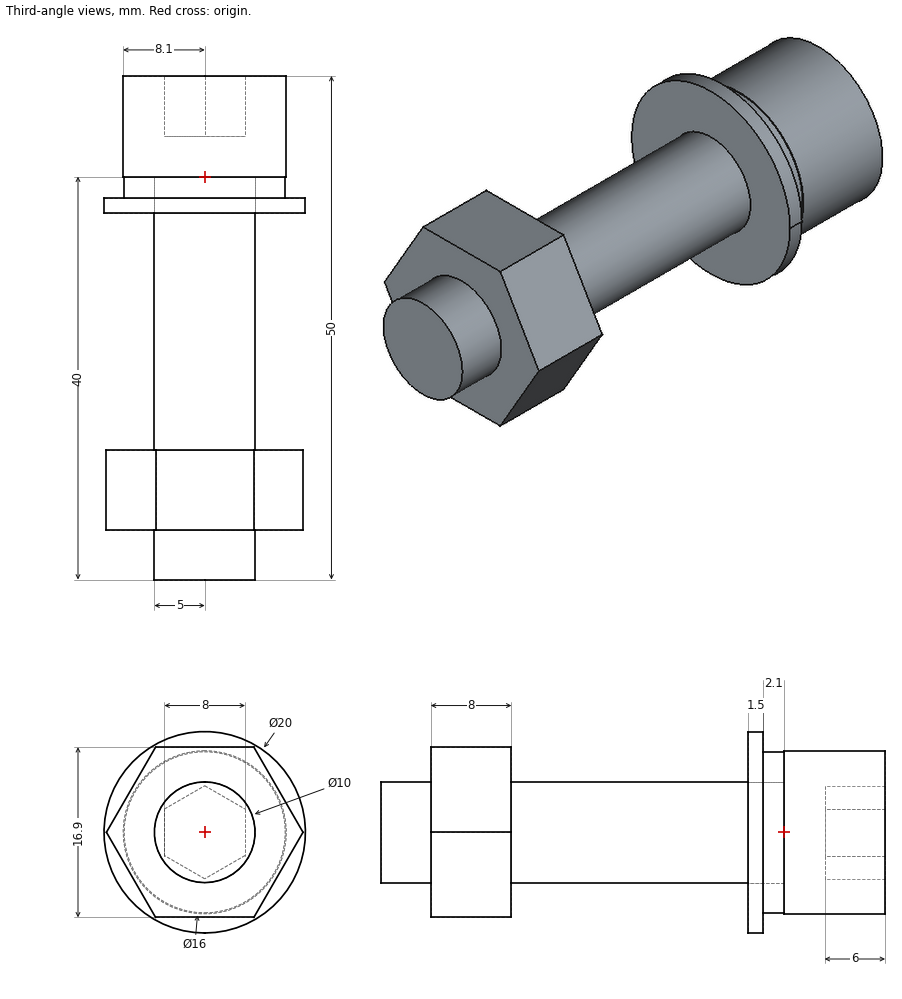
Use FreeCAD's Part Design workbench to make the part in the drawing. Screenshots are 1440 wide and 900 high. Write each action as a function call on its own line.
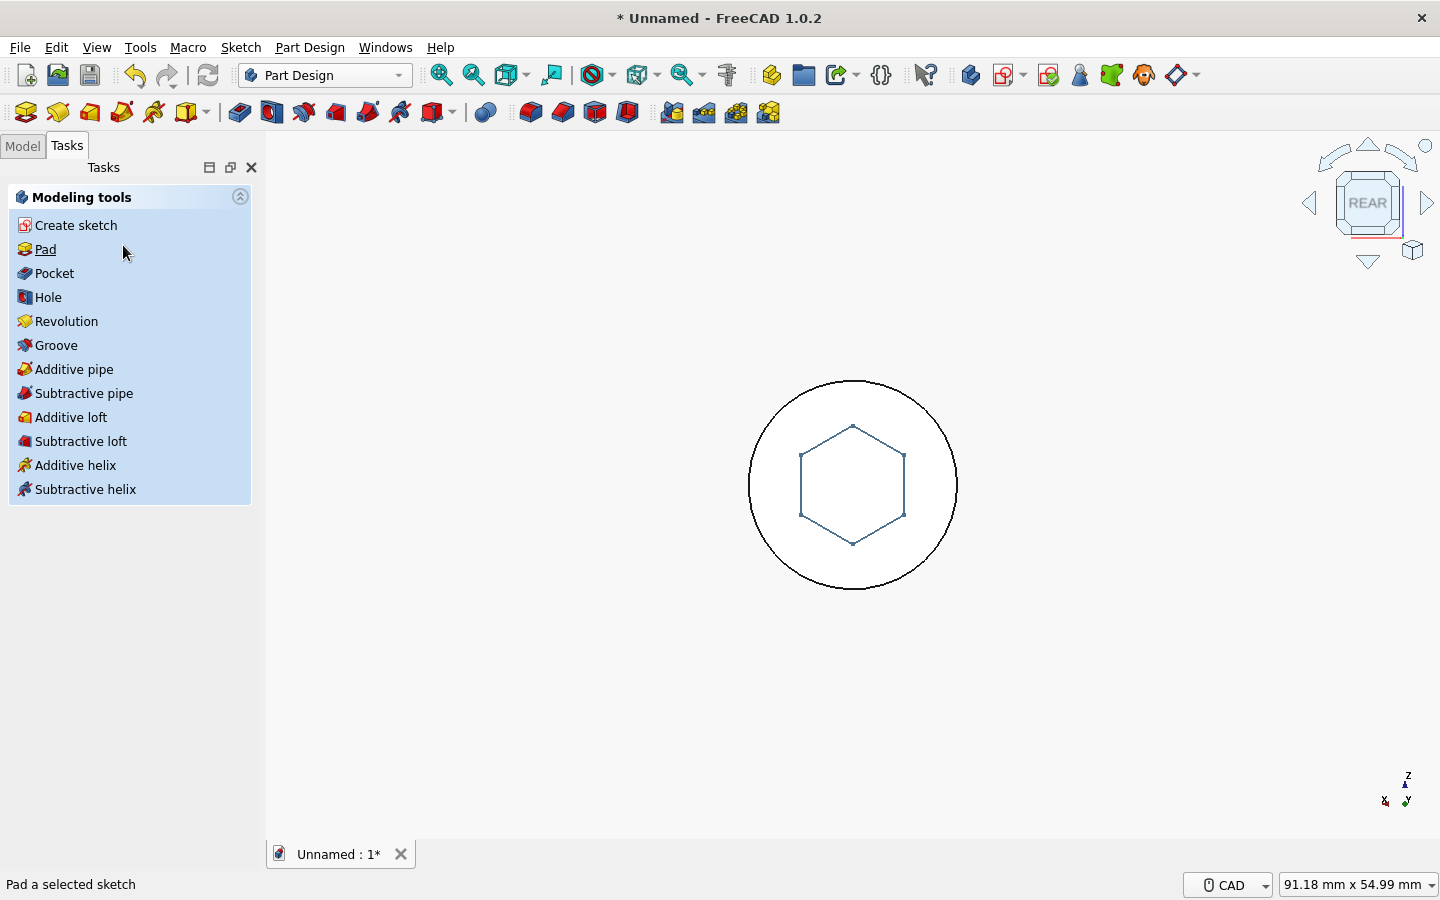
click(240, 112)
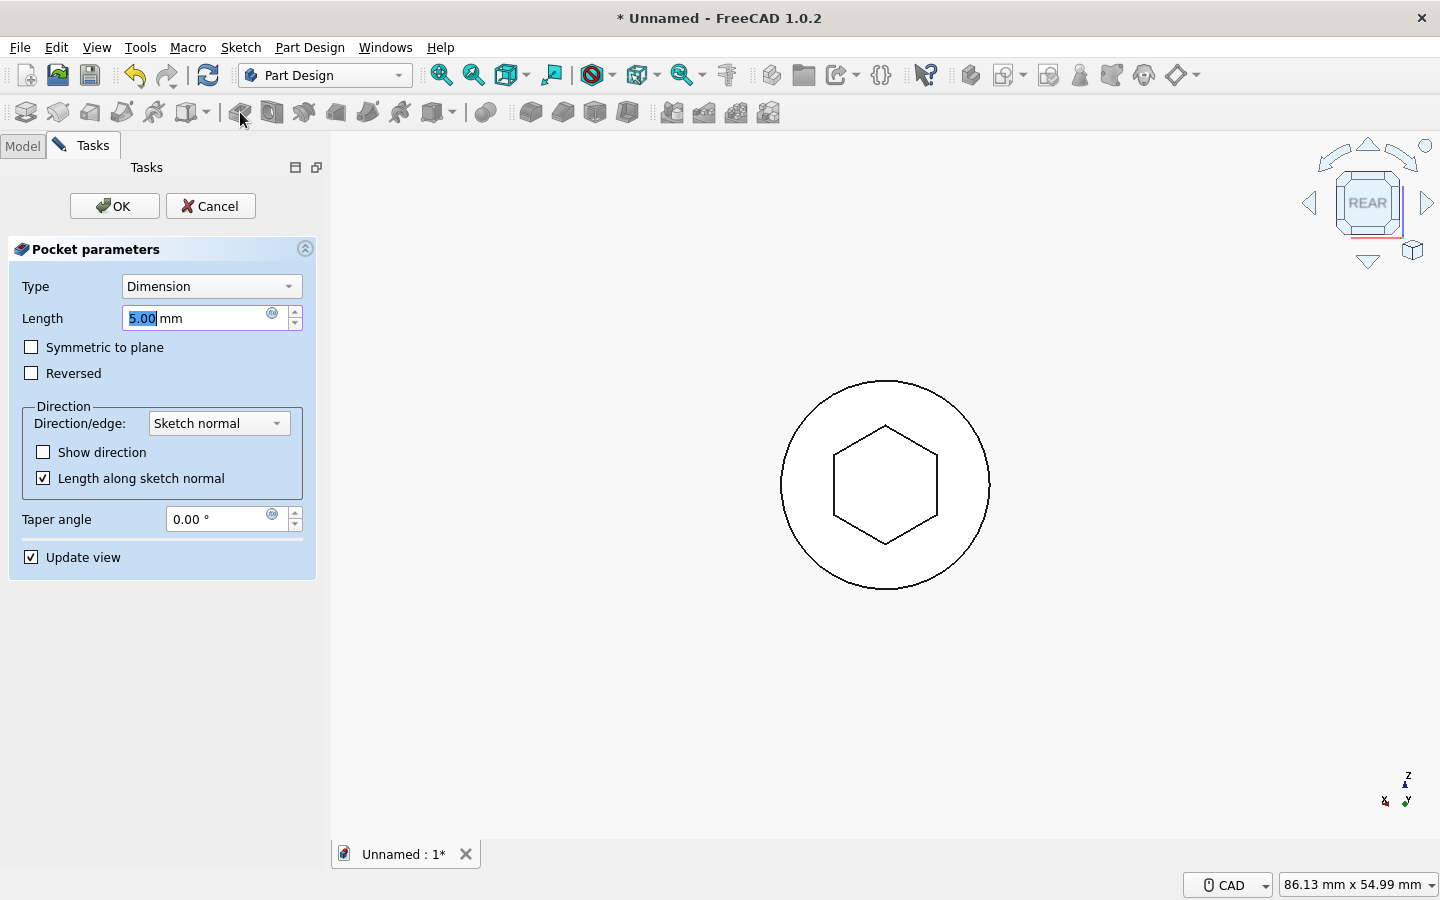
text(6)
key(Tab)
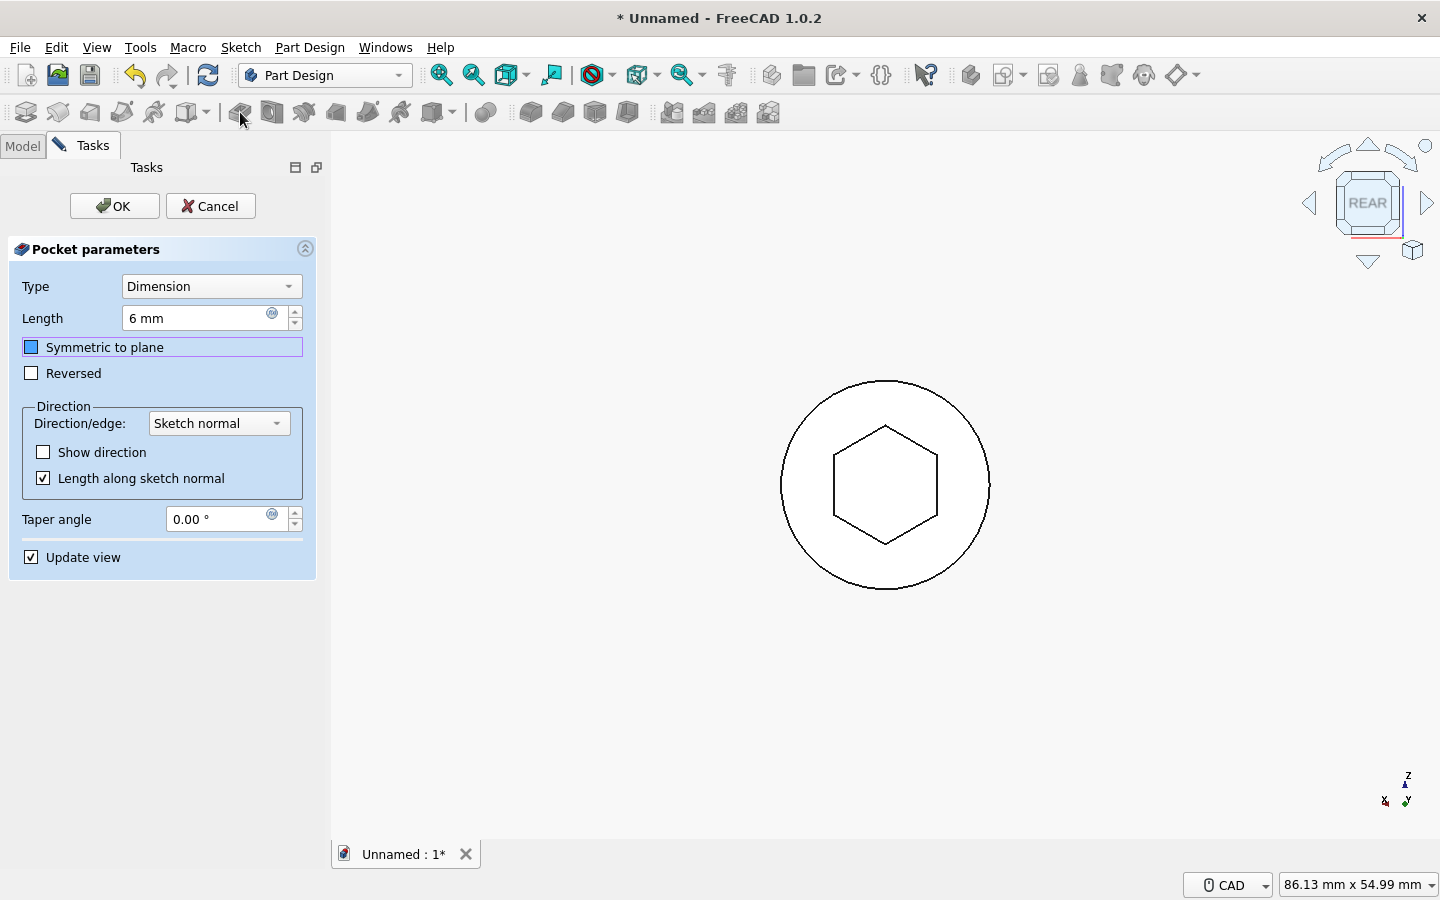
click(115, 206)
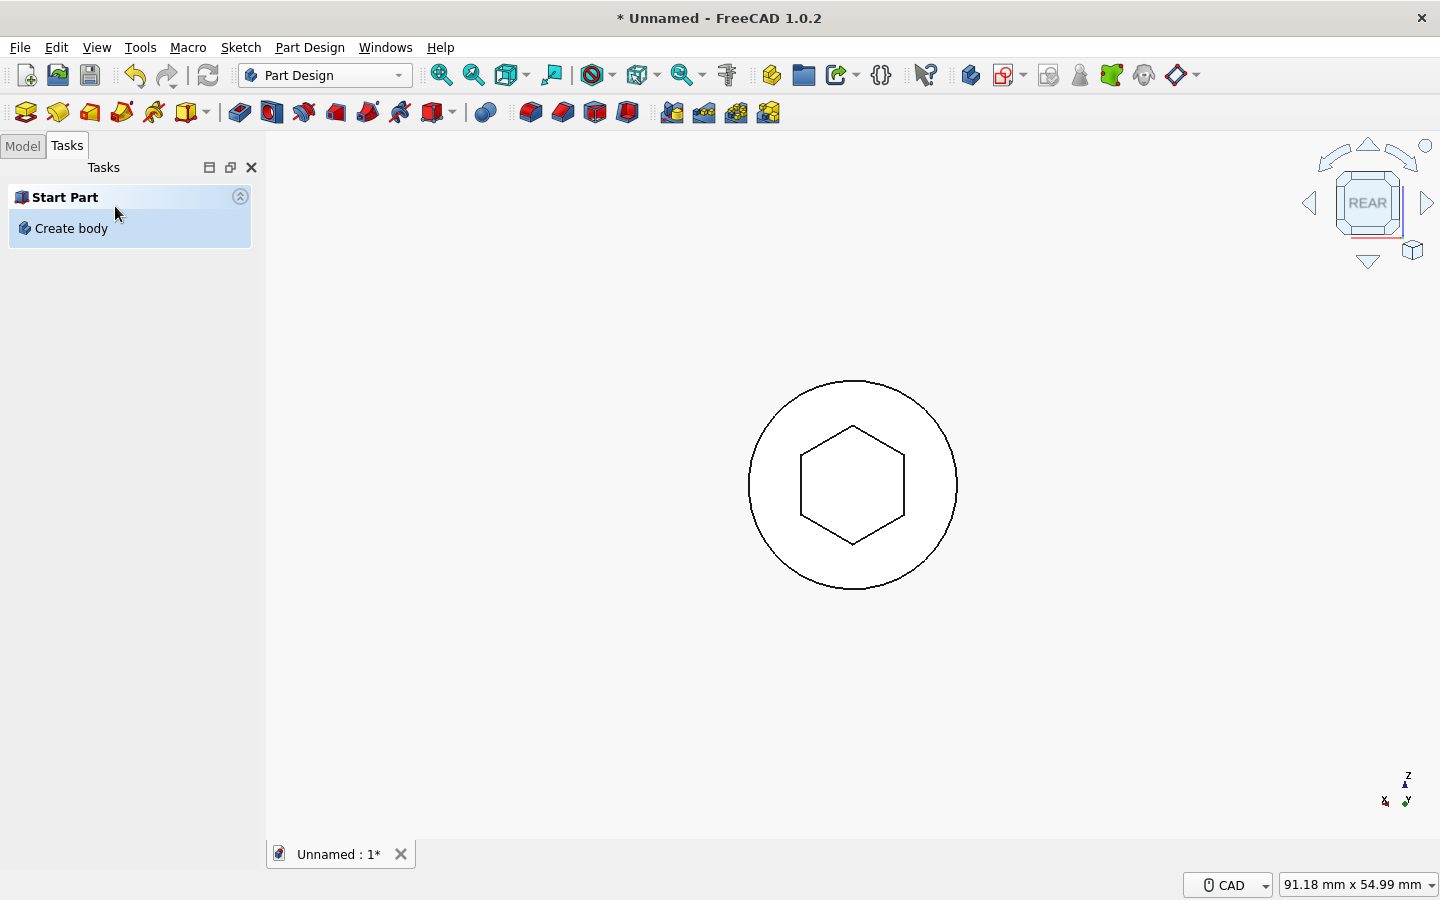
click(442, 76)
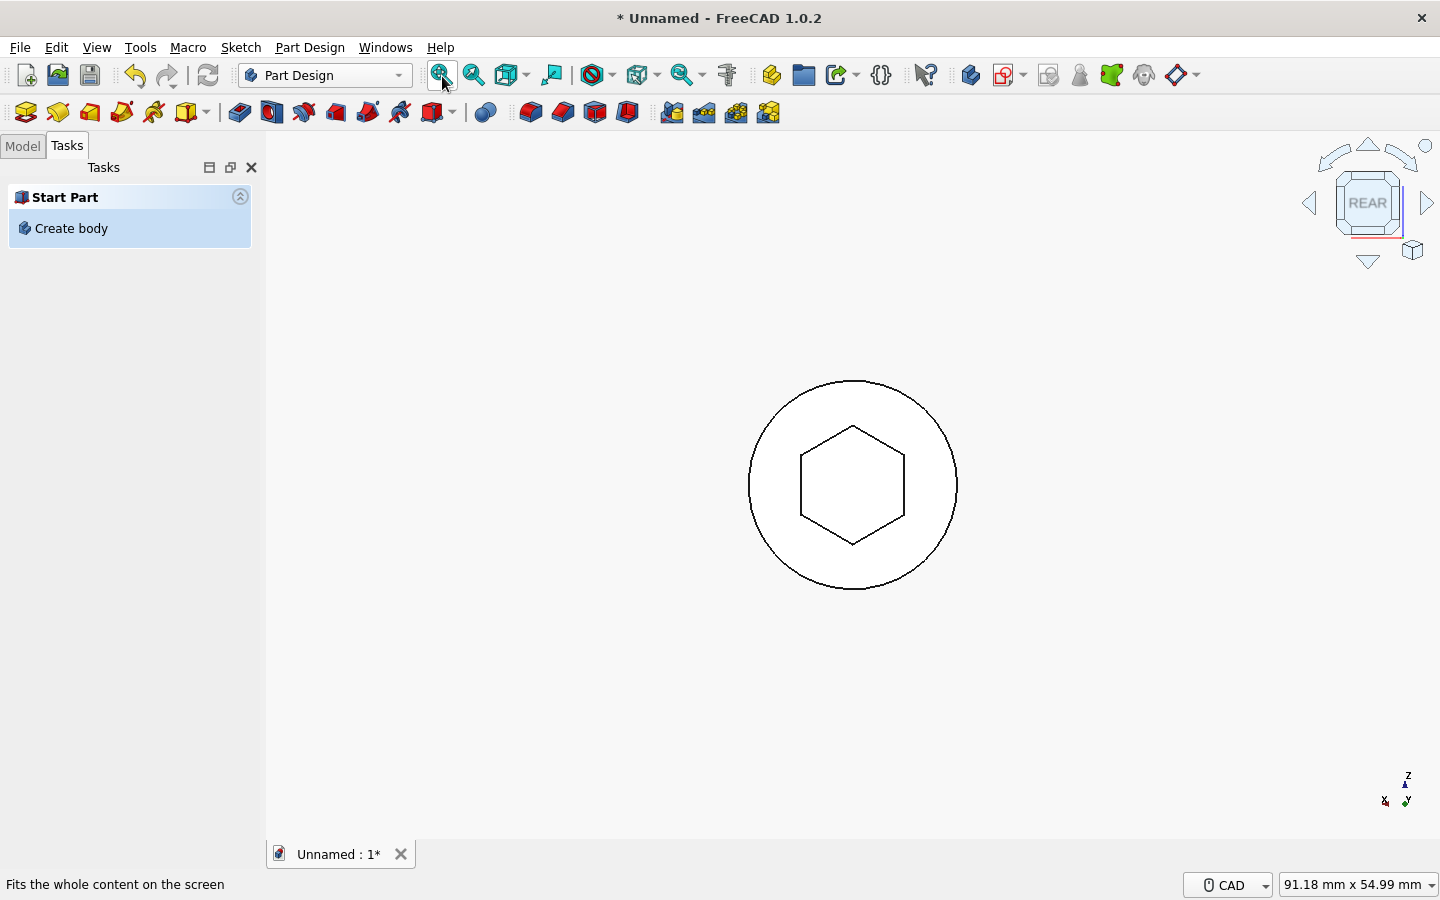
click(23, 145)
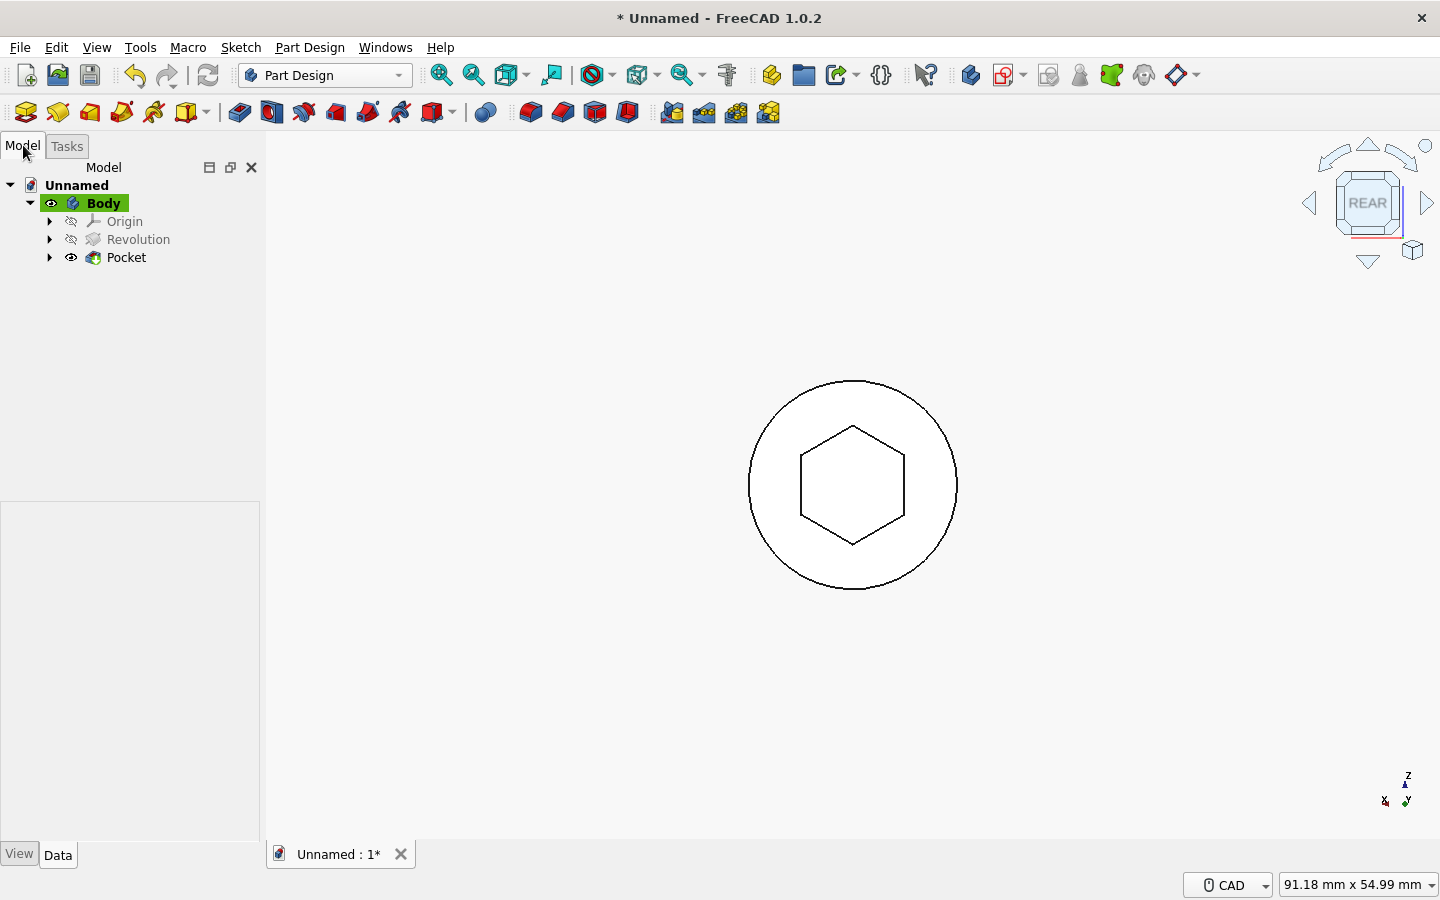
click(50, 221)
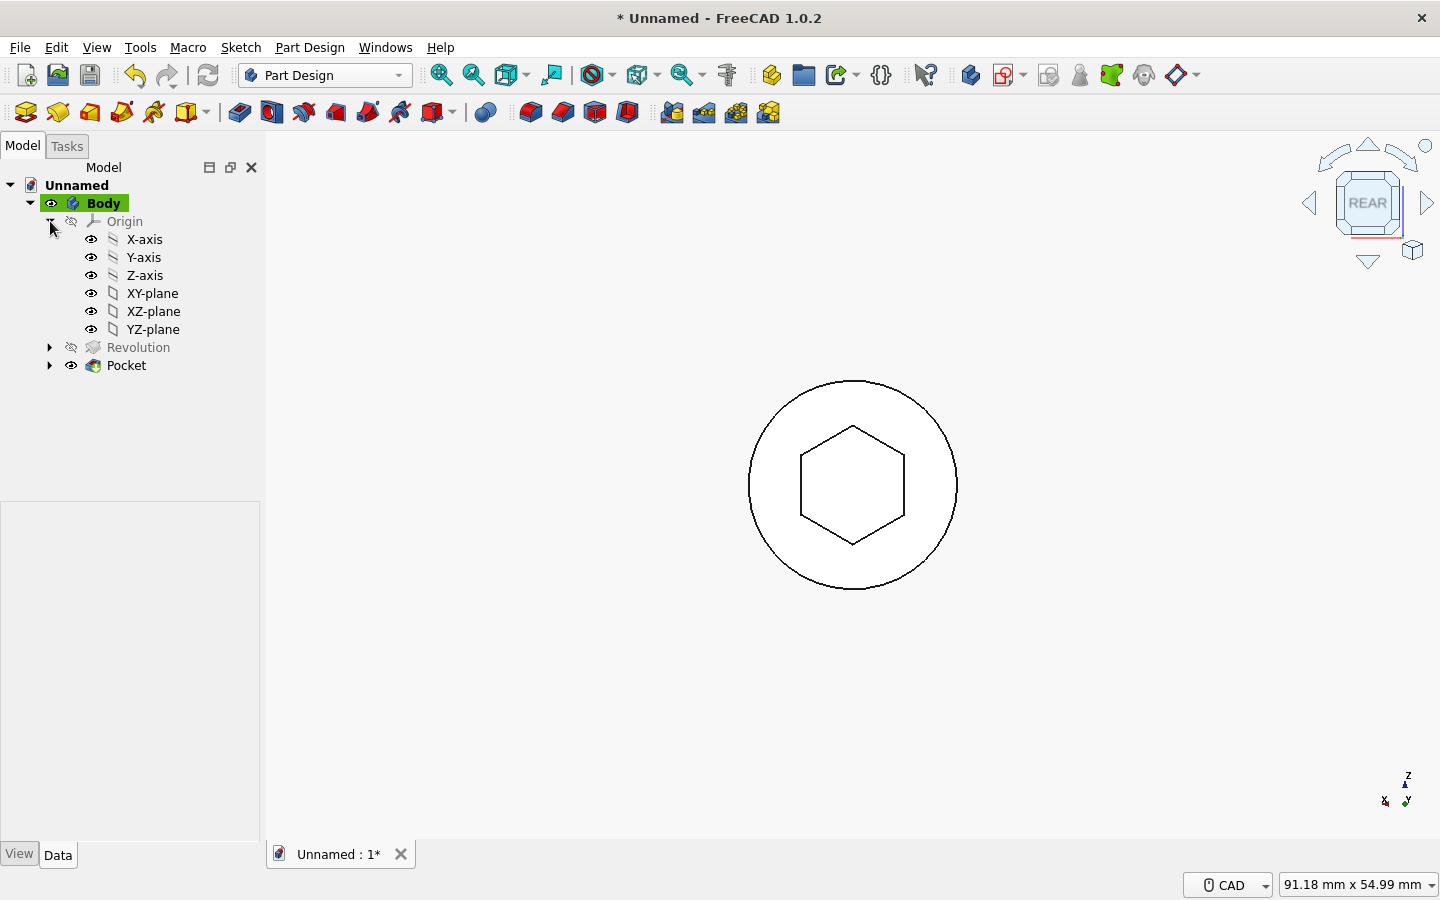
click(136, 311)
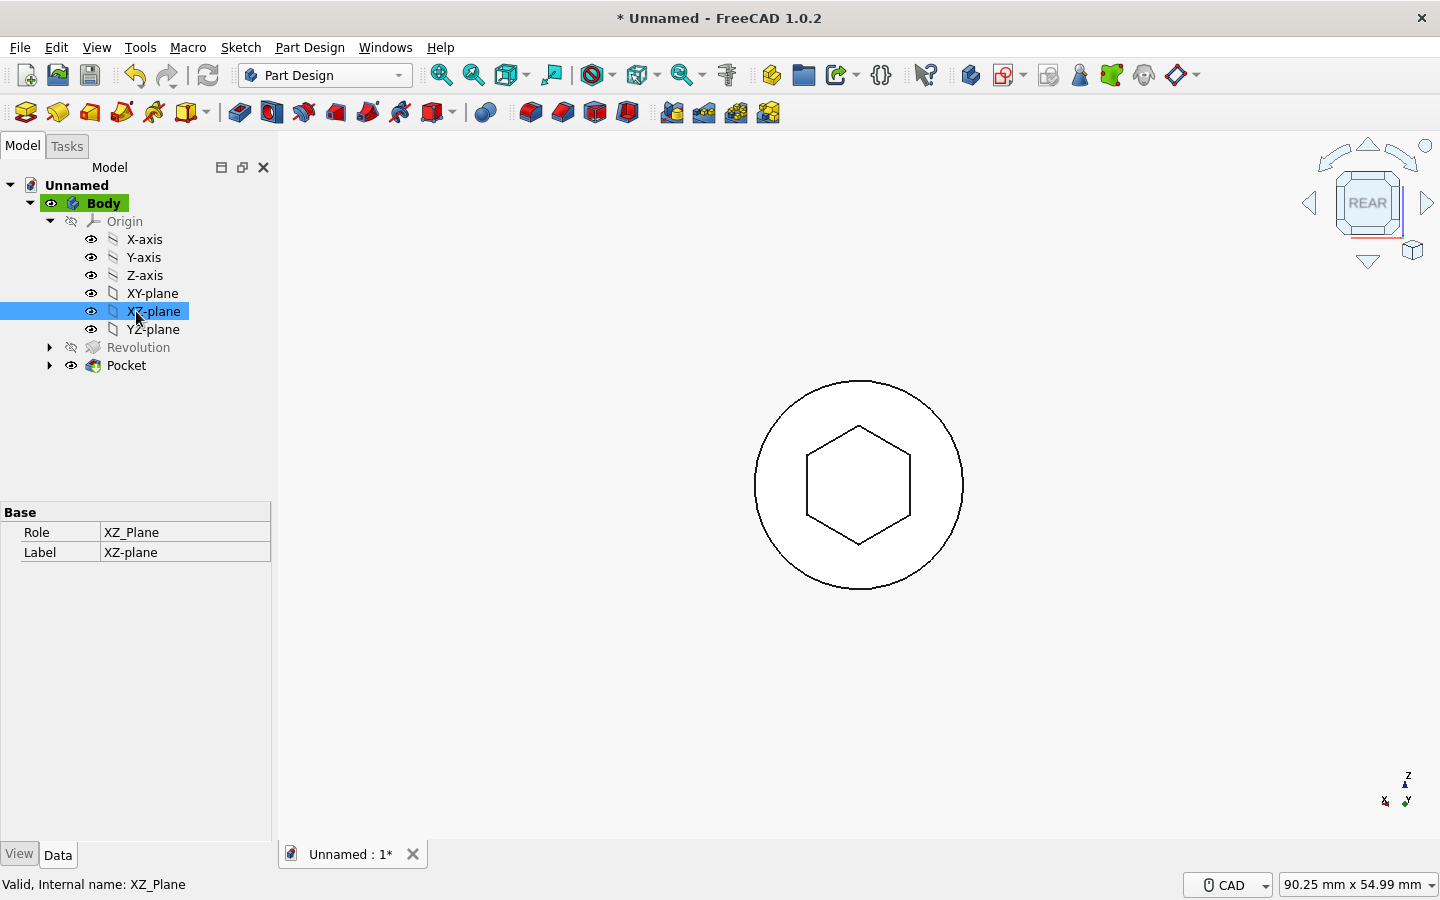
click(1176, 76)